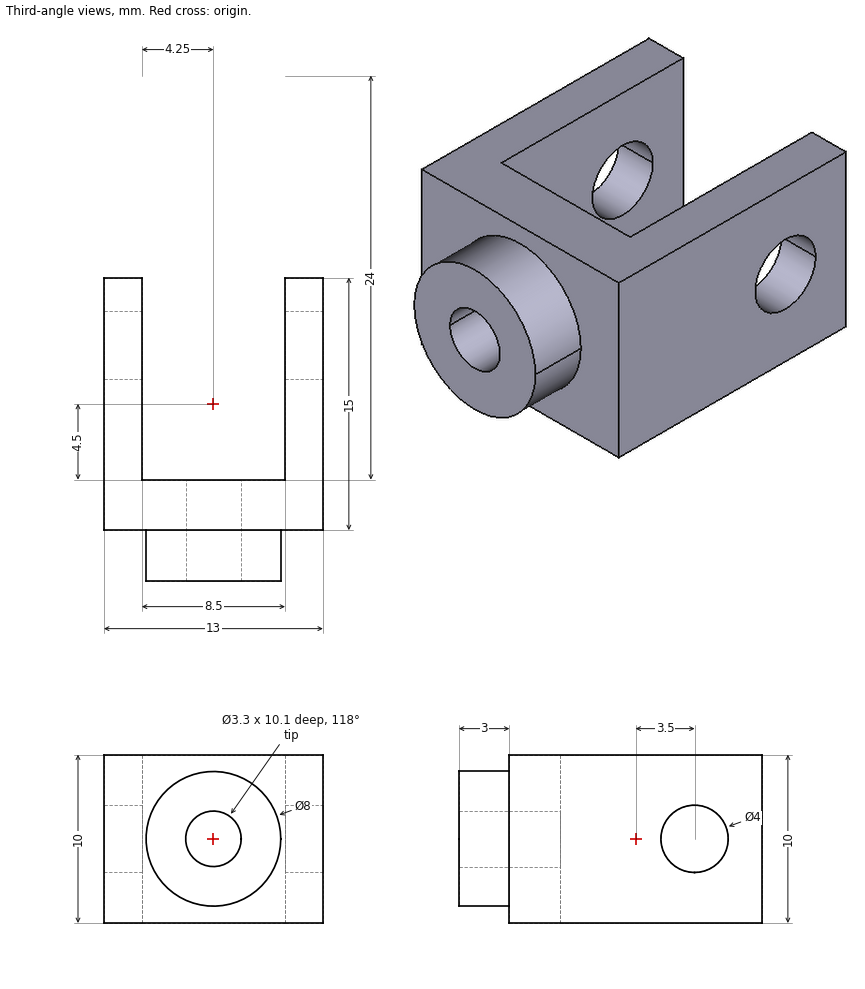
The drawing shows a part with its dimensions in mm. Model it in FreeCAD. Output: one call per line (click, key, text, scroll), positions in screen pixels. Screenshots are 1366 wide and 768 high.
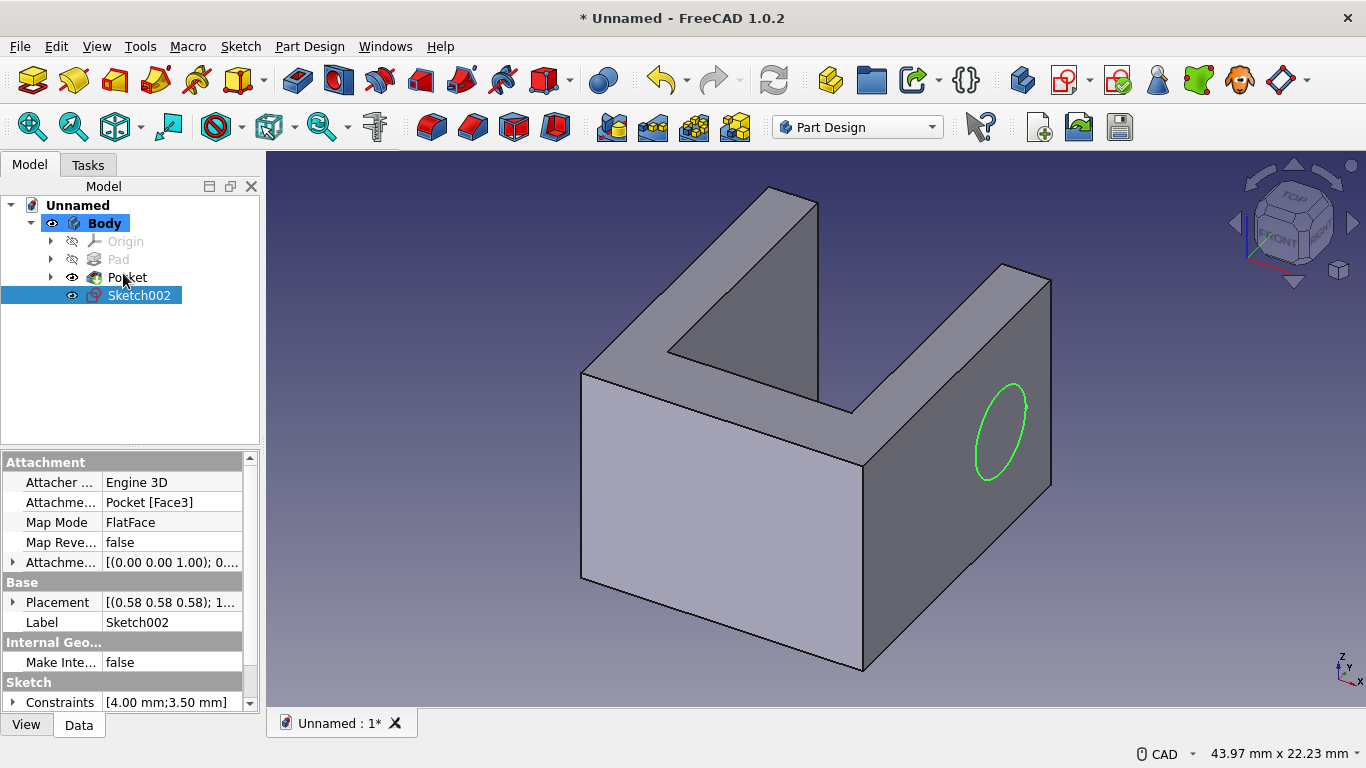
click(298, 80)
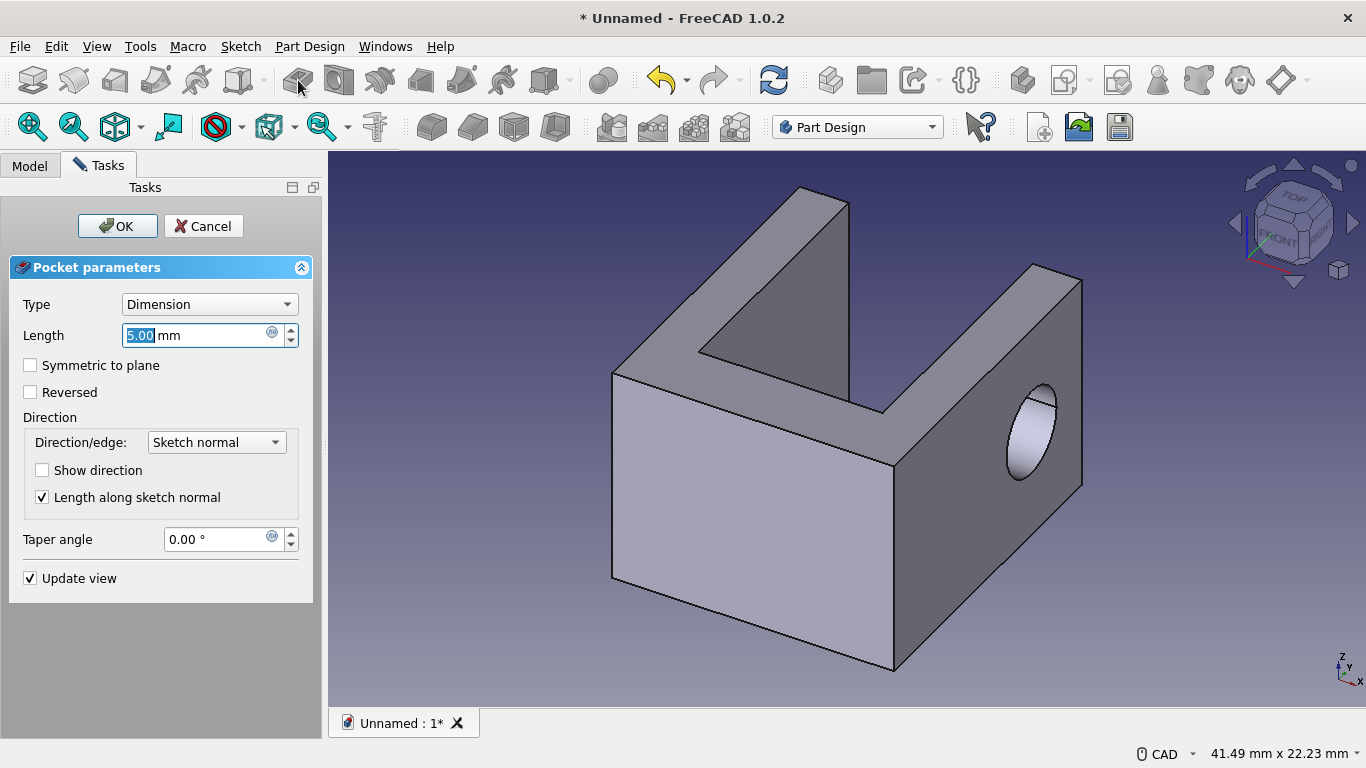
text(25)
key(Tab)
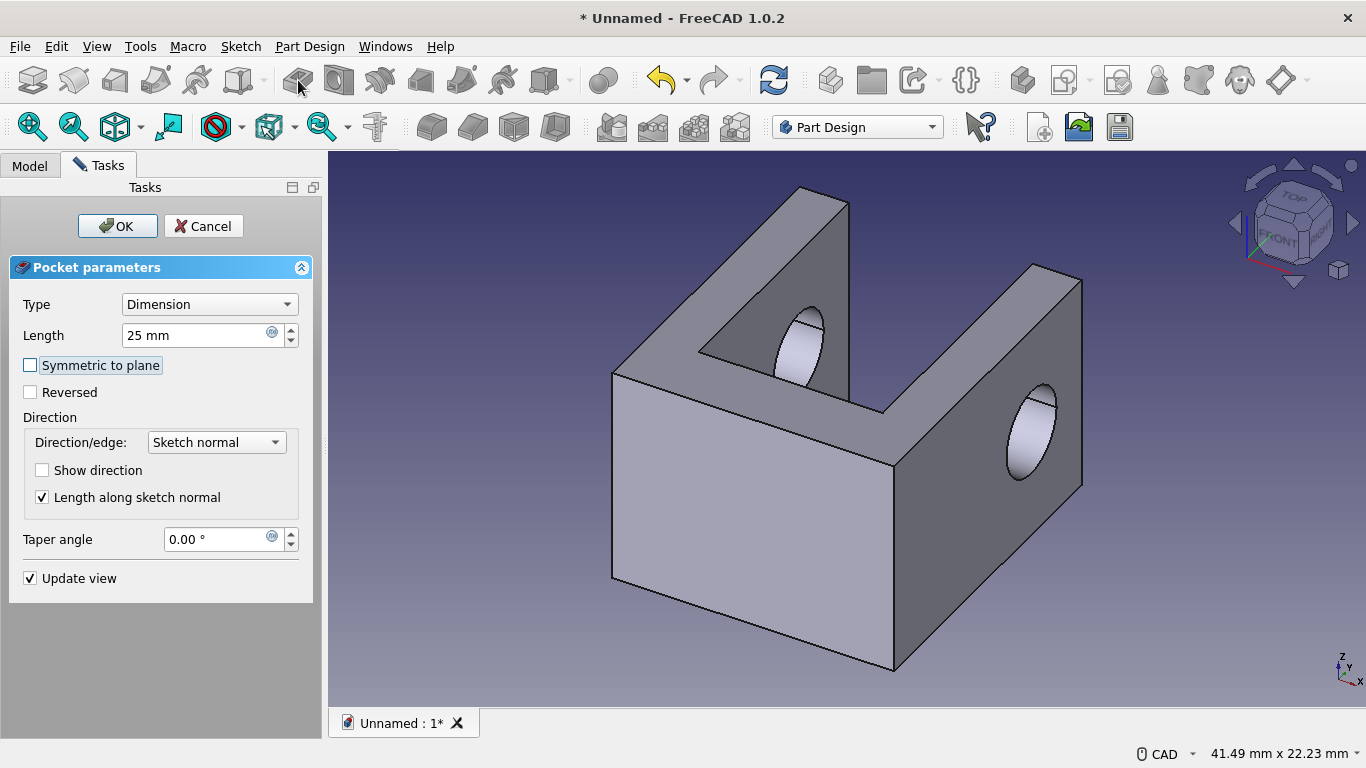
click(118, 226)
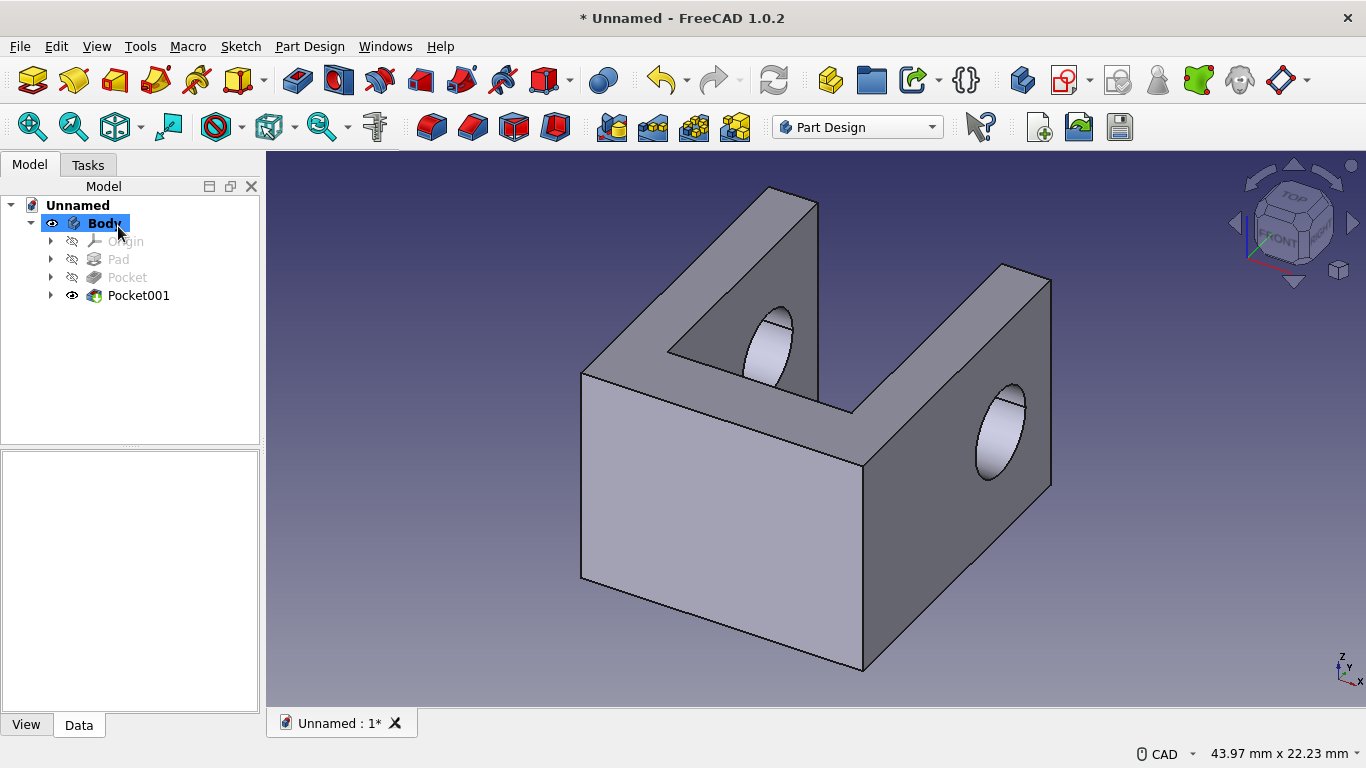
click(722, 521)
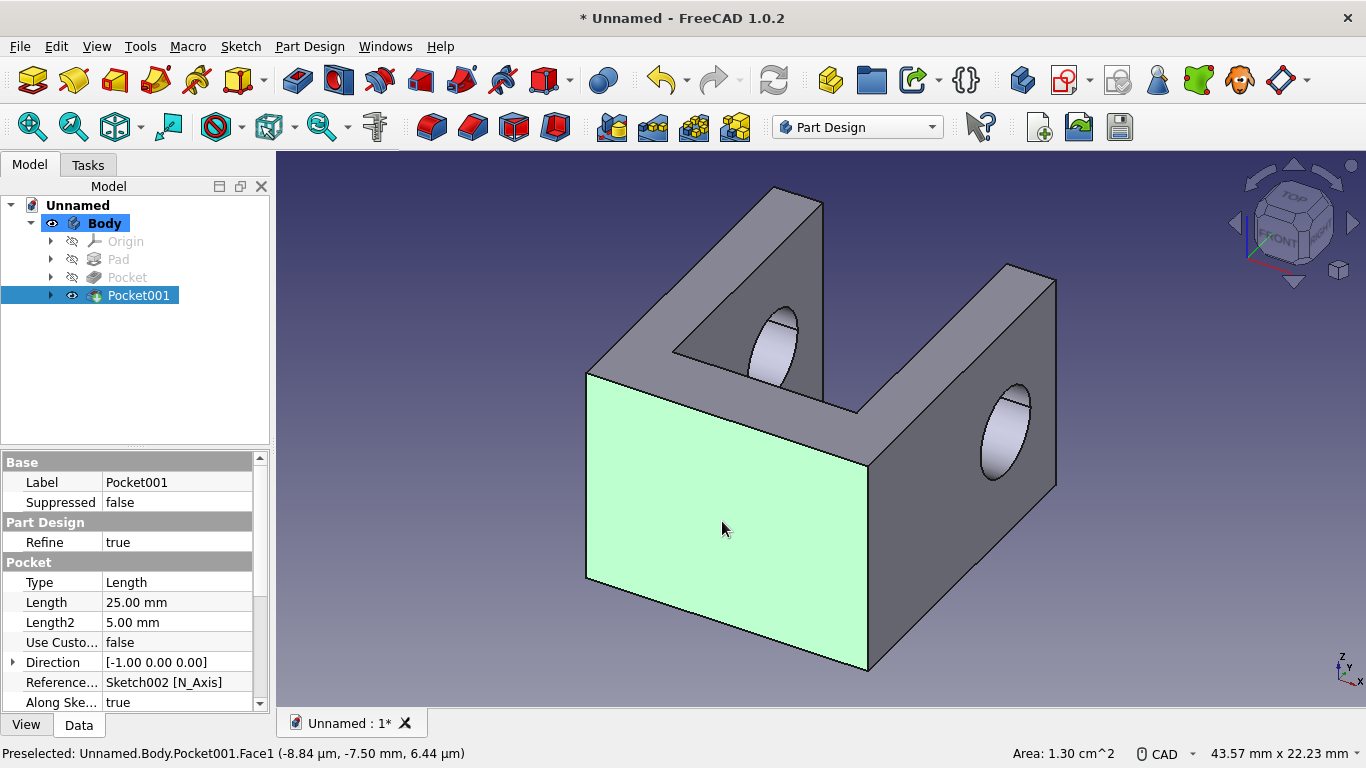
click(1064, 80)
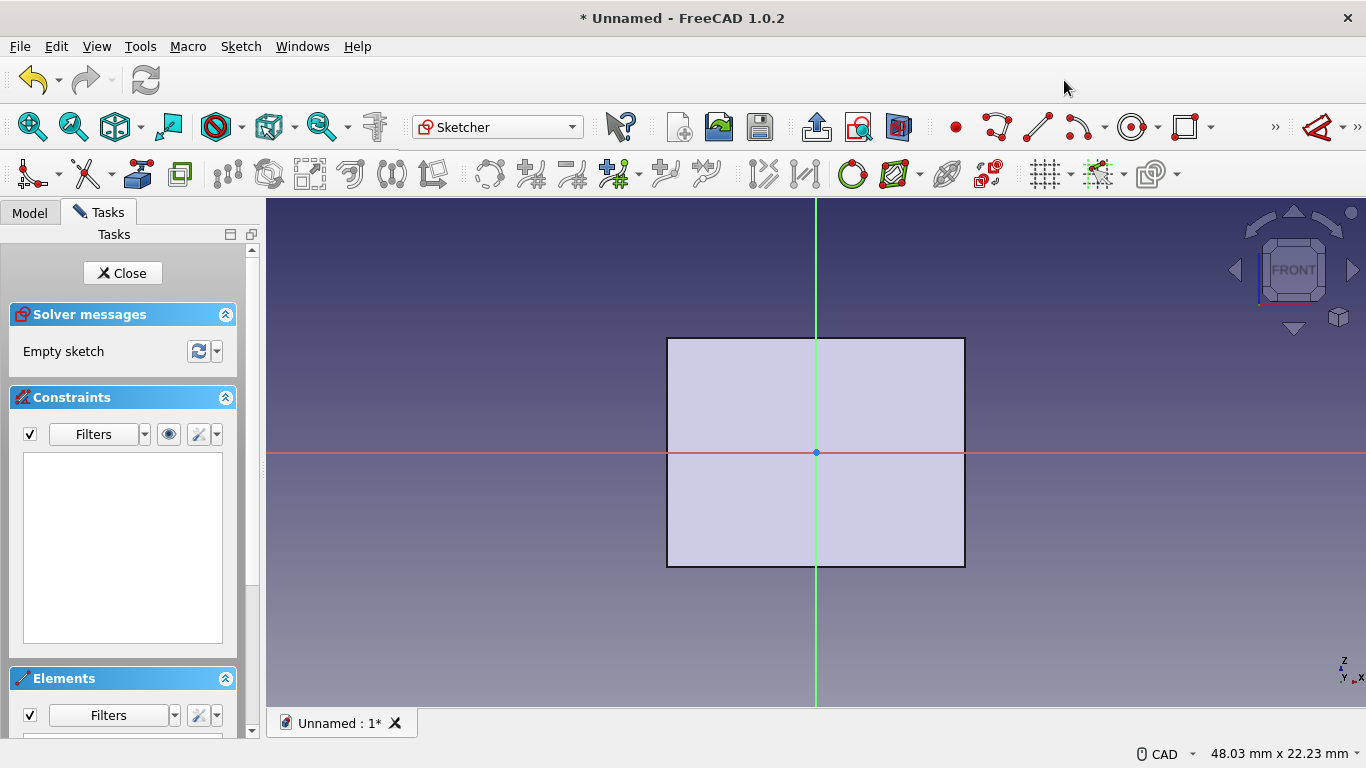
scroll(899, 452, up, 3)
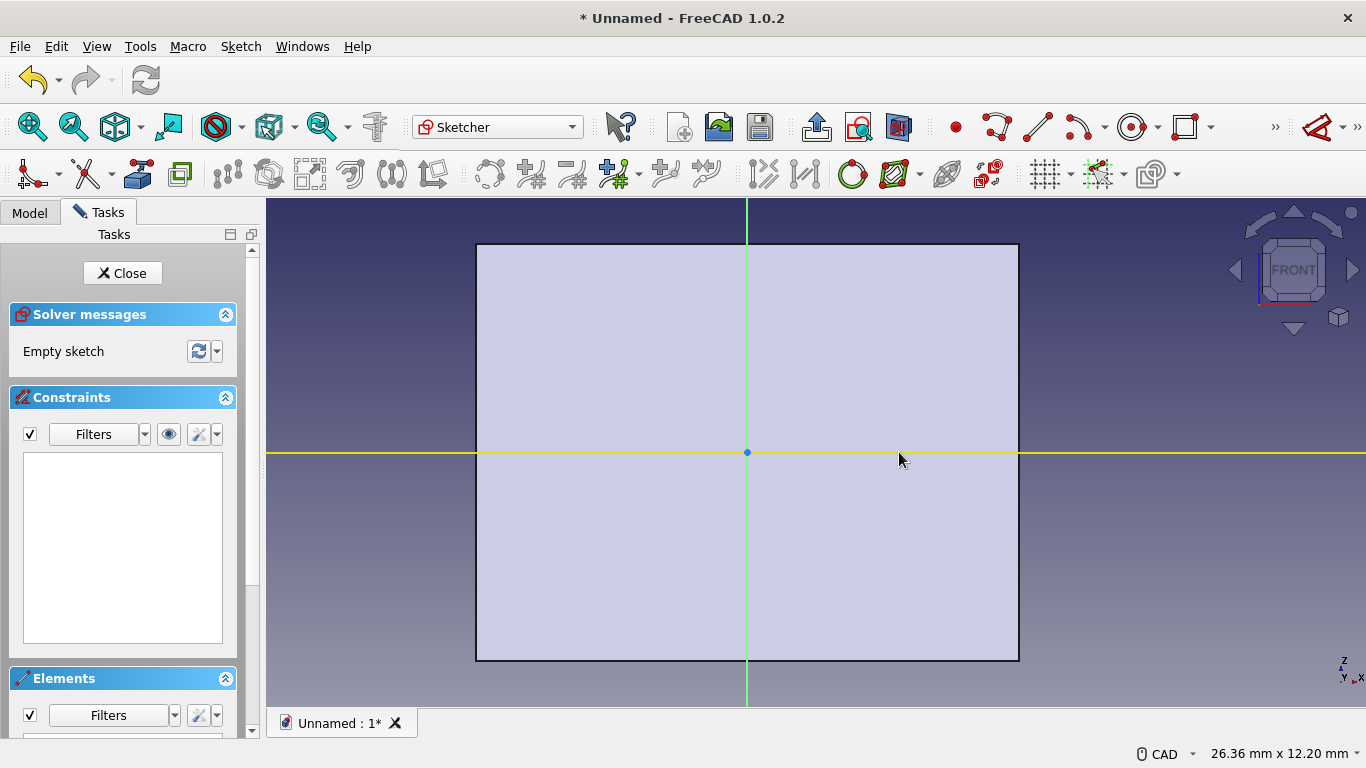
key(g)
key(c)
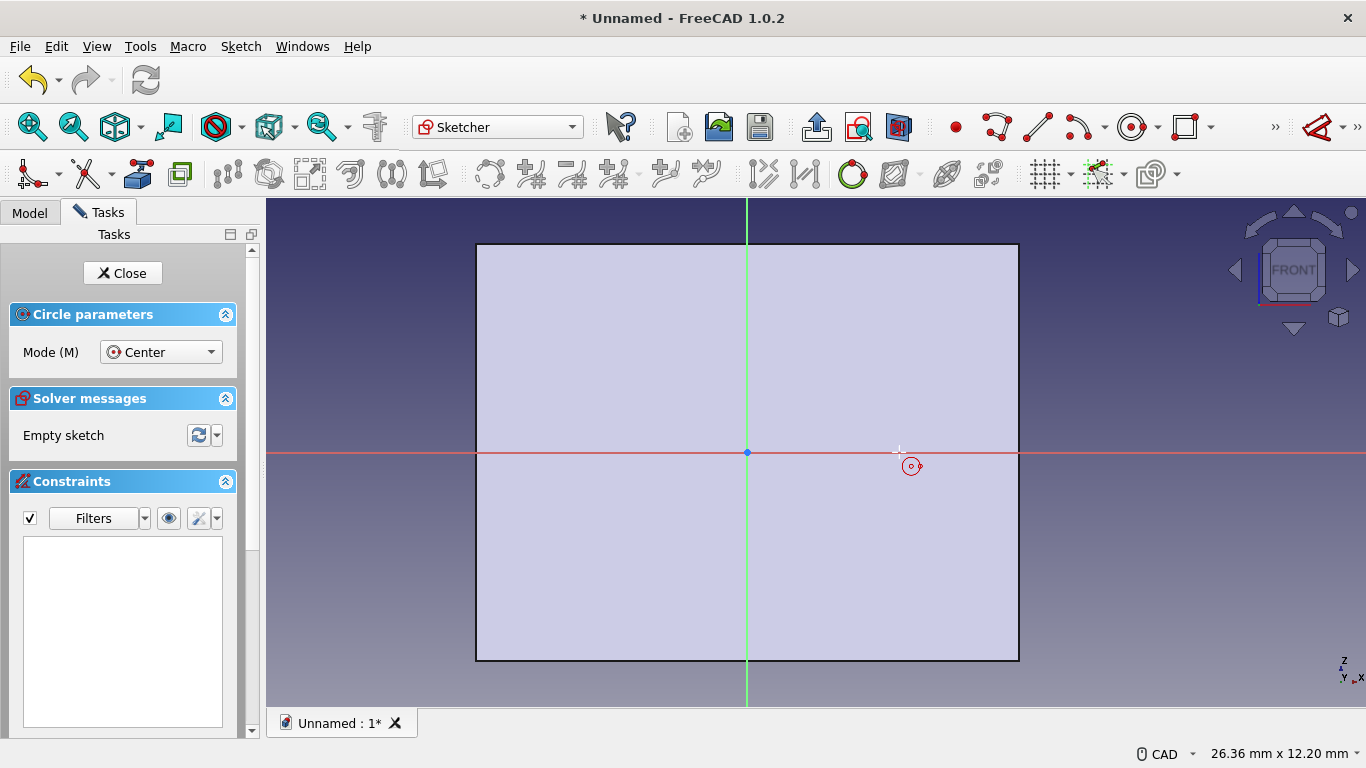
click(747, 452)
move(865, 334)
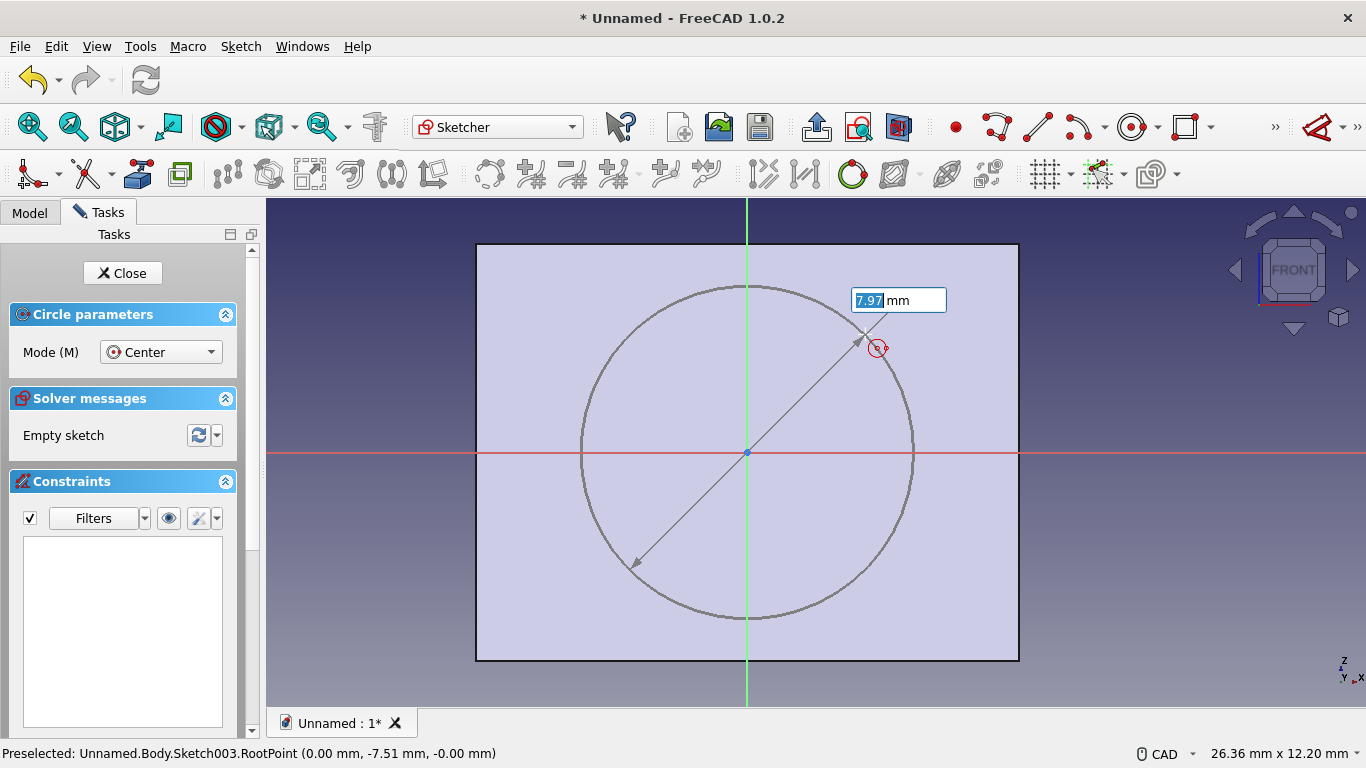
text(8)
key(Return)
key(Escape)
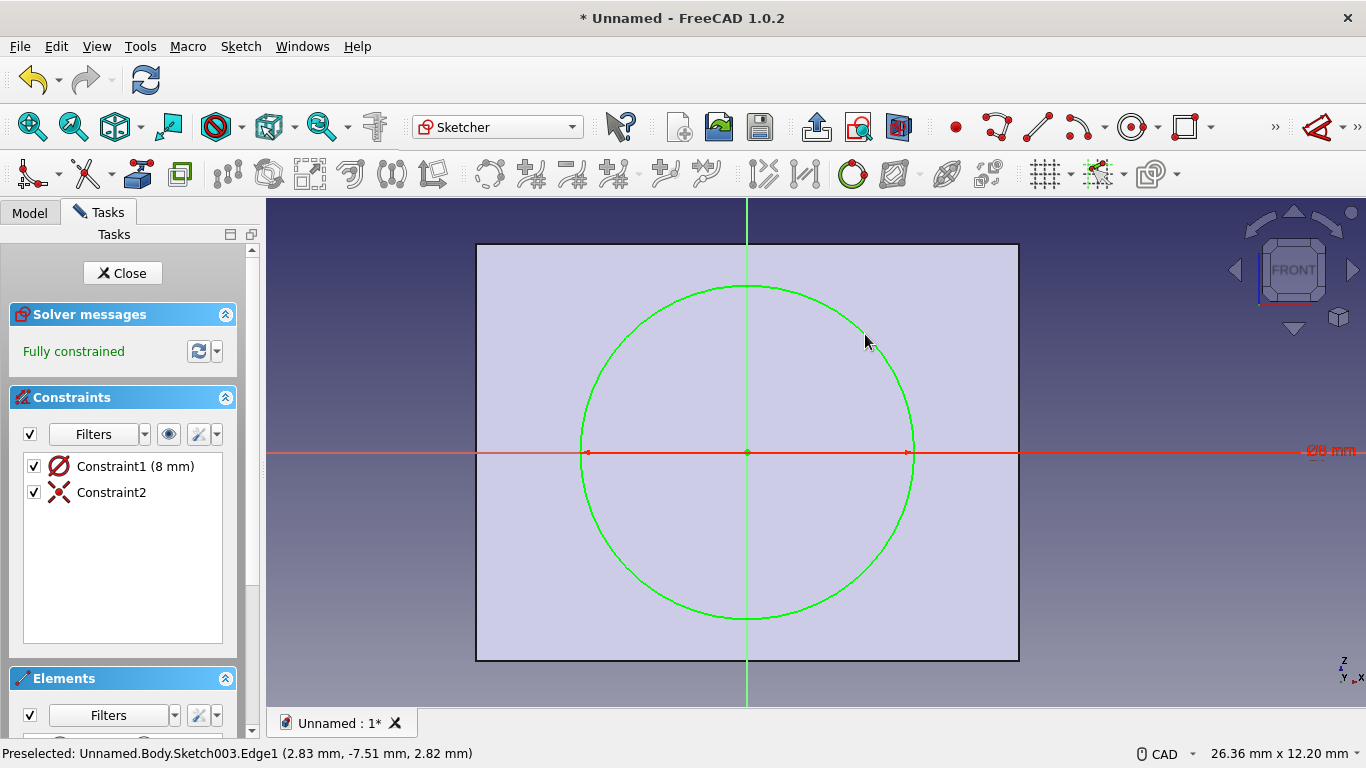
click(123, 273)